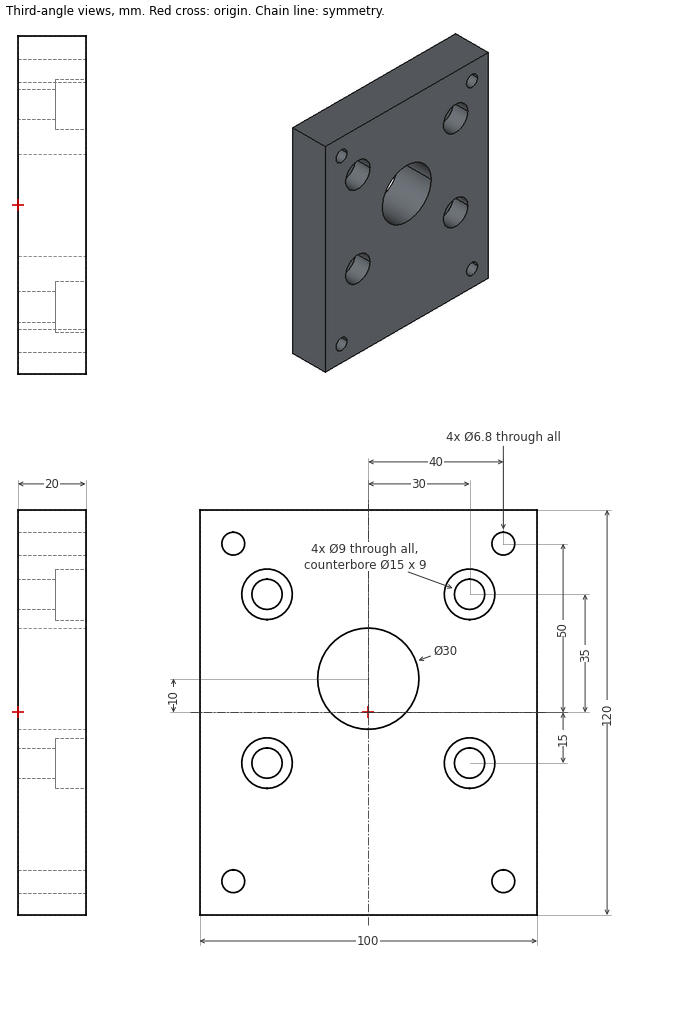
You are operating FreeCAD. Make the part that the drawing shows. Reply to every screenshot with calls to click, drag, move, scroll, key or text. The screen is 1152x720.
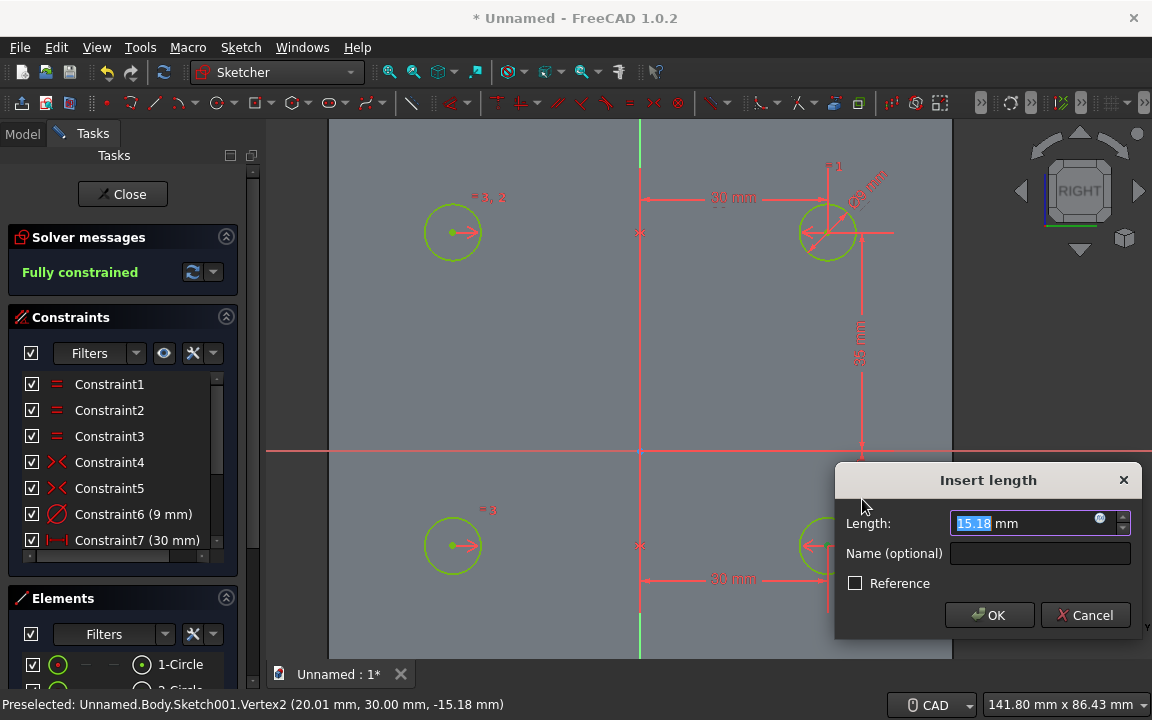
text(15)
key(Return)
key(Escape)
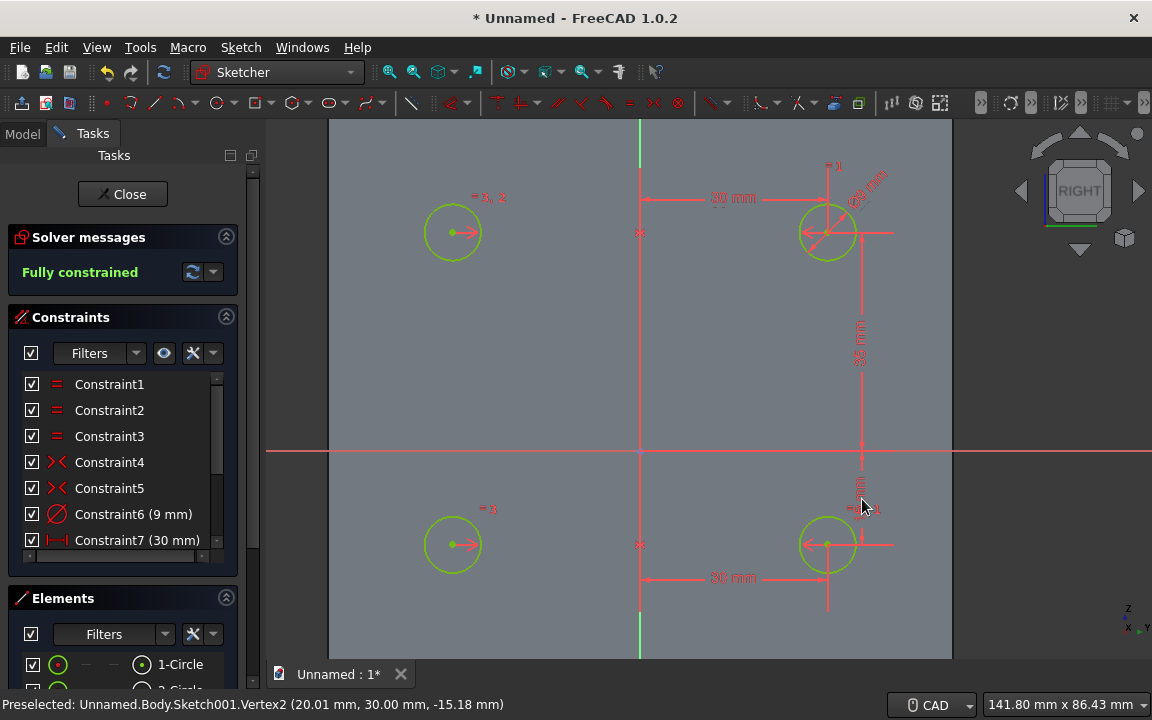
click(123, 194)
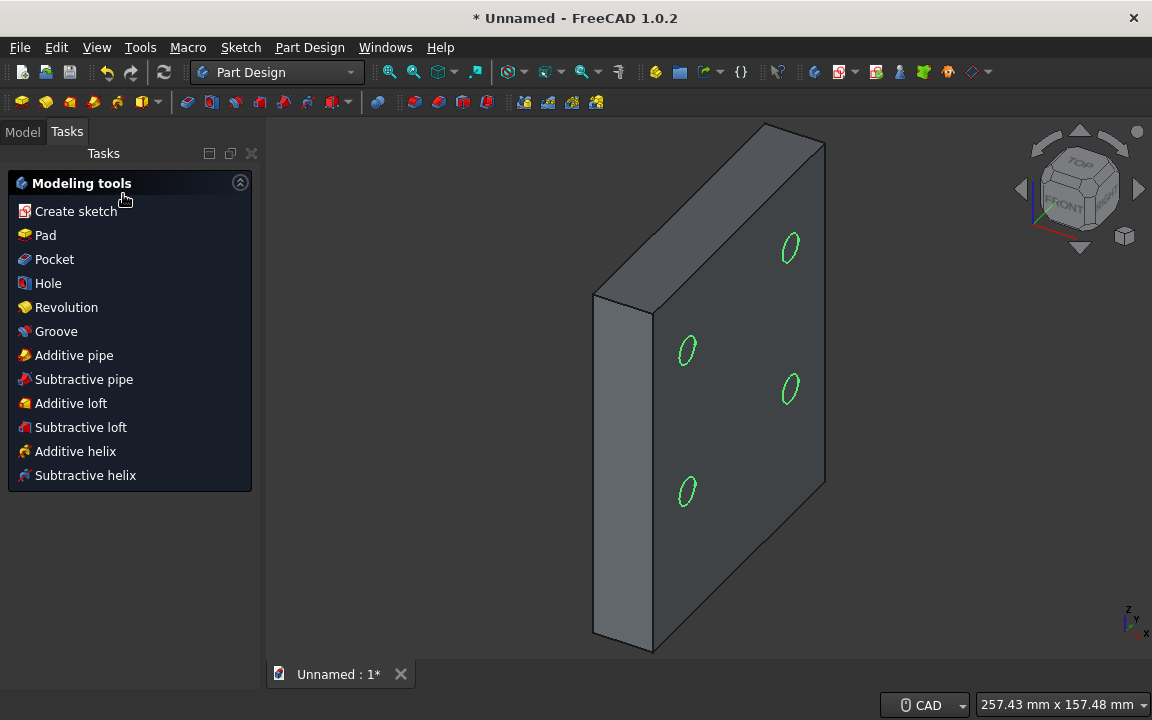
click(212, 102)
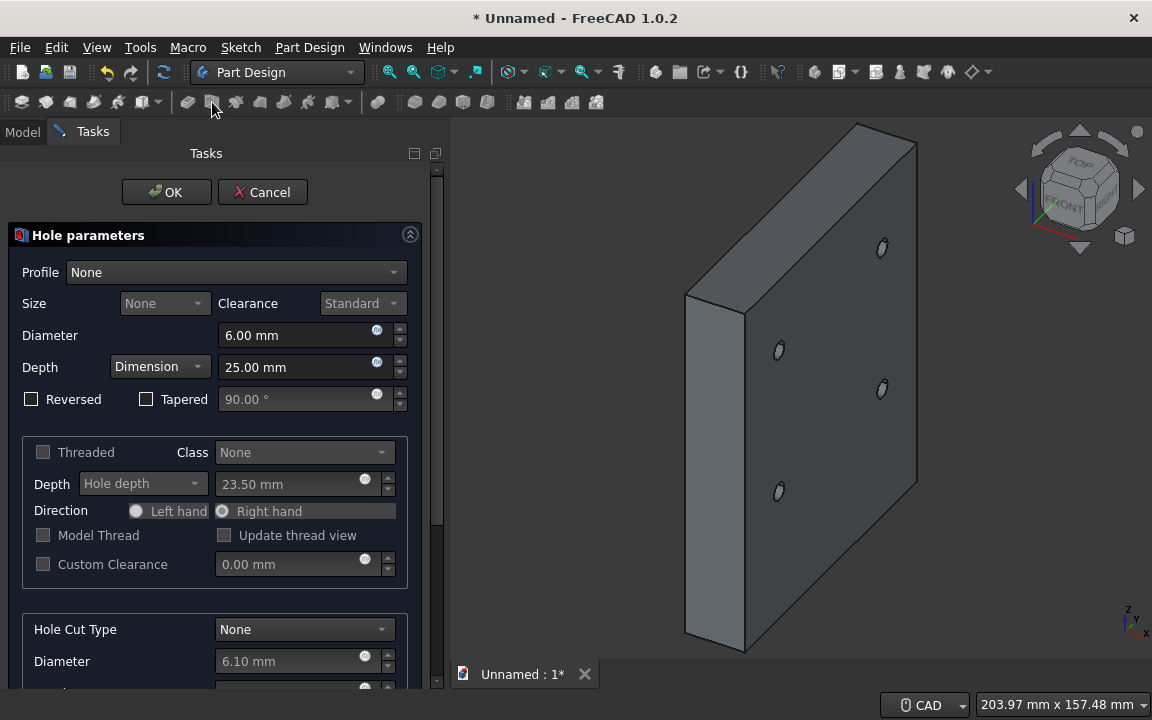
triple_click(305, 335)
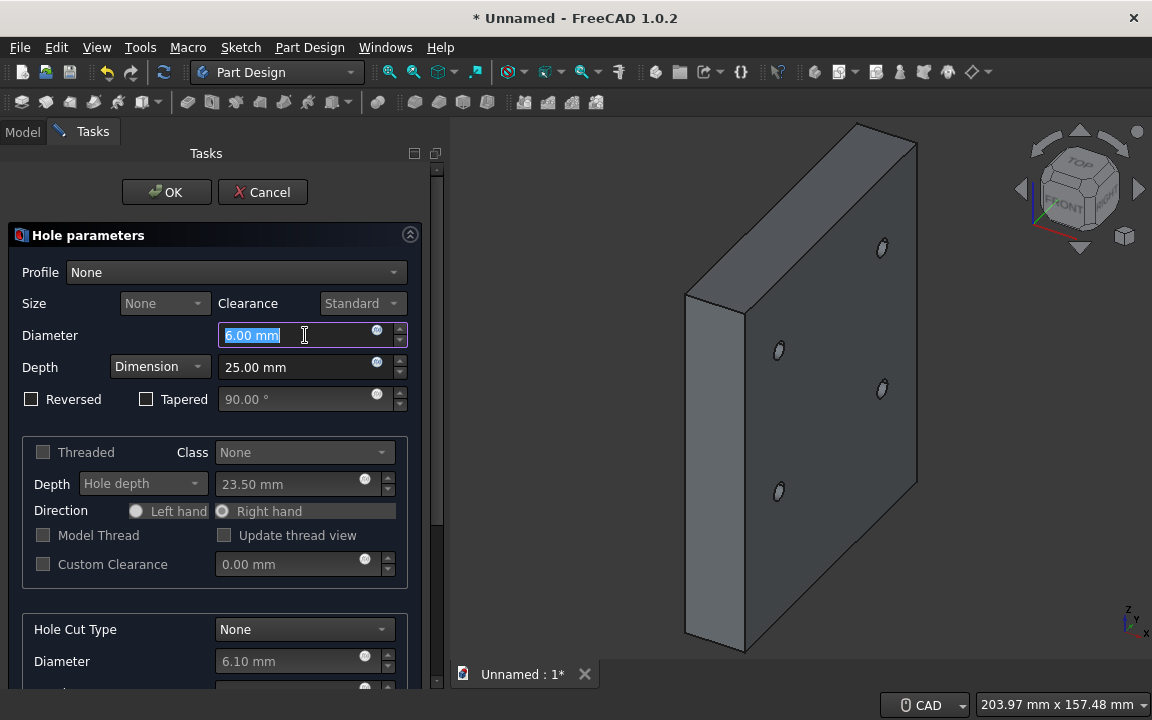
text(9)
key(Tab)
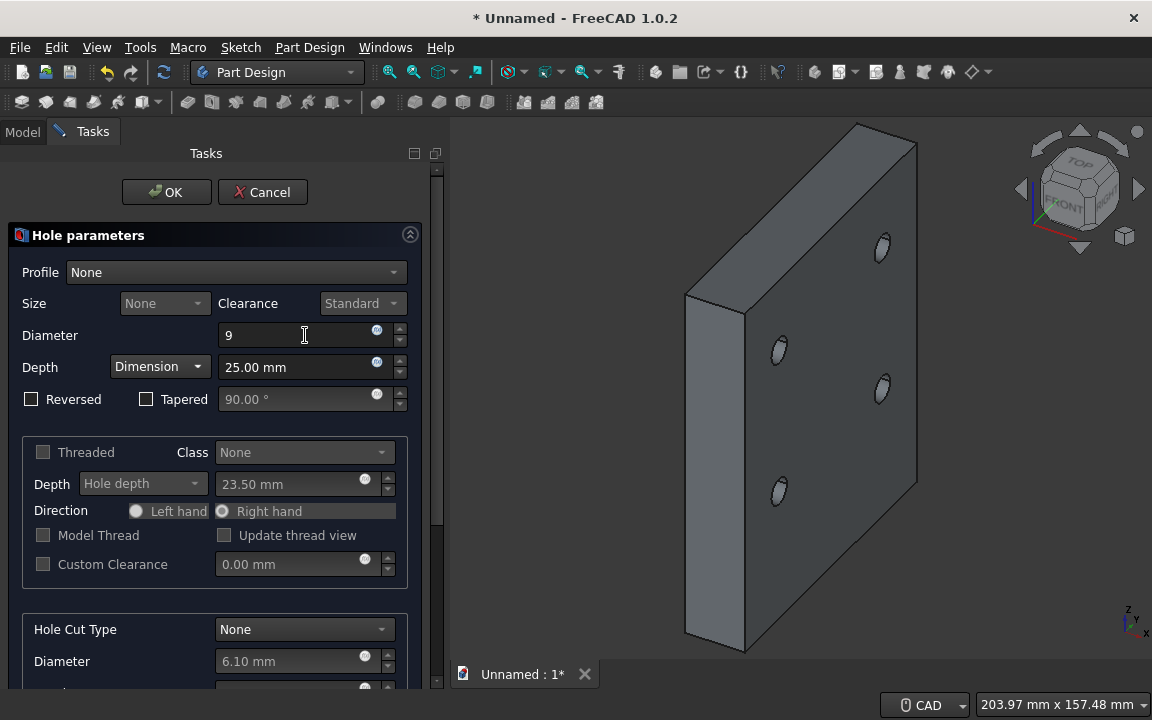
click(161, 366)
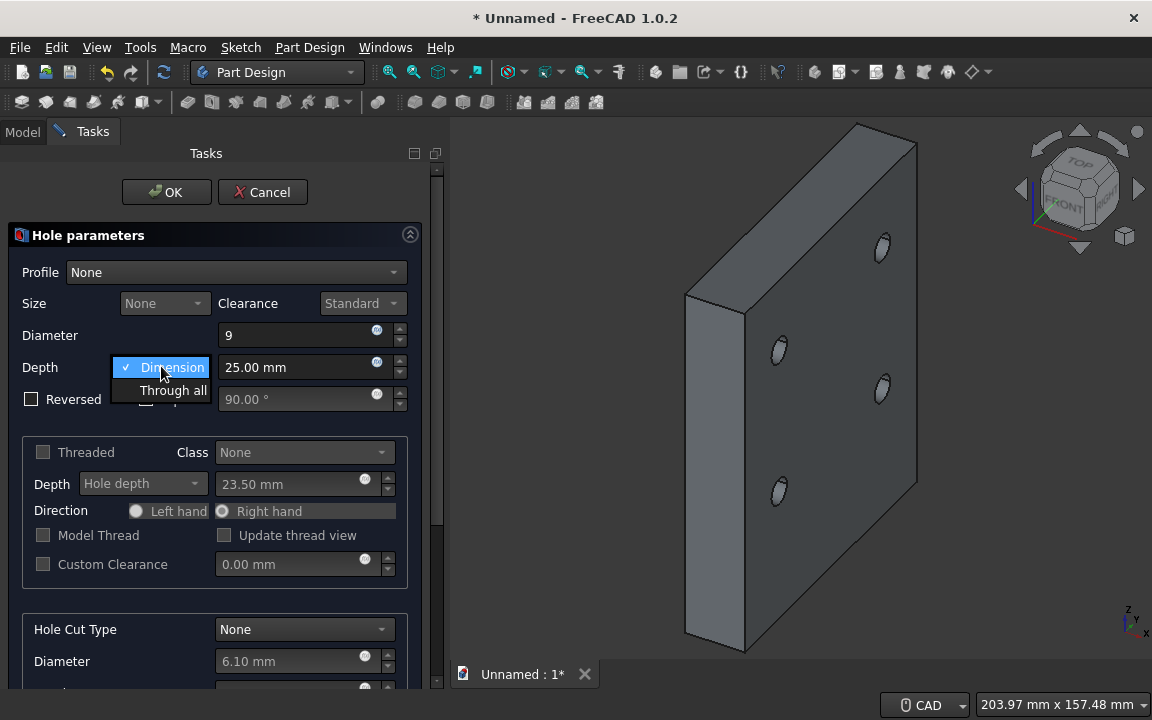
click(160, 390)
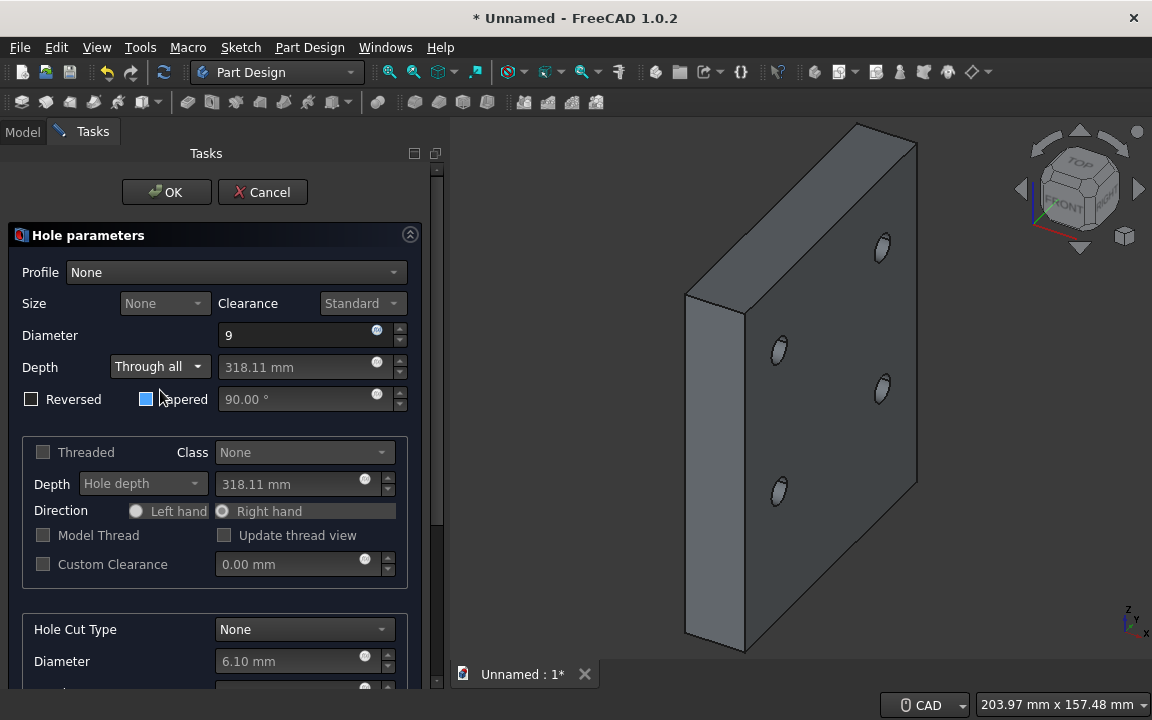
click(306, 630)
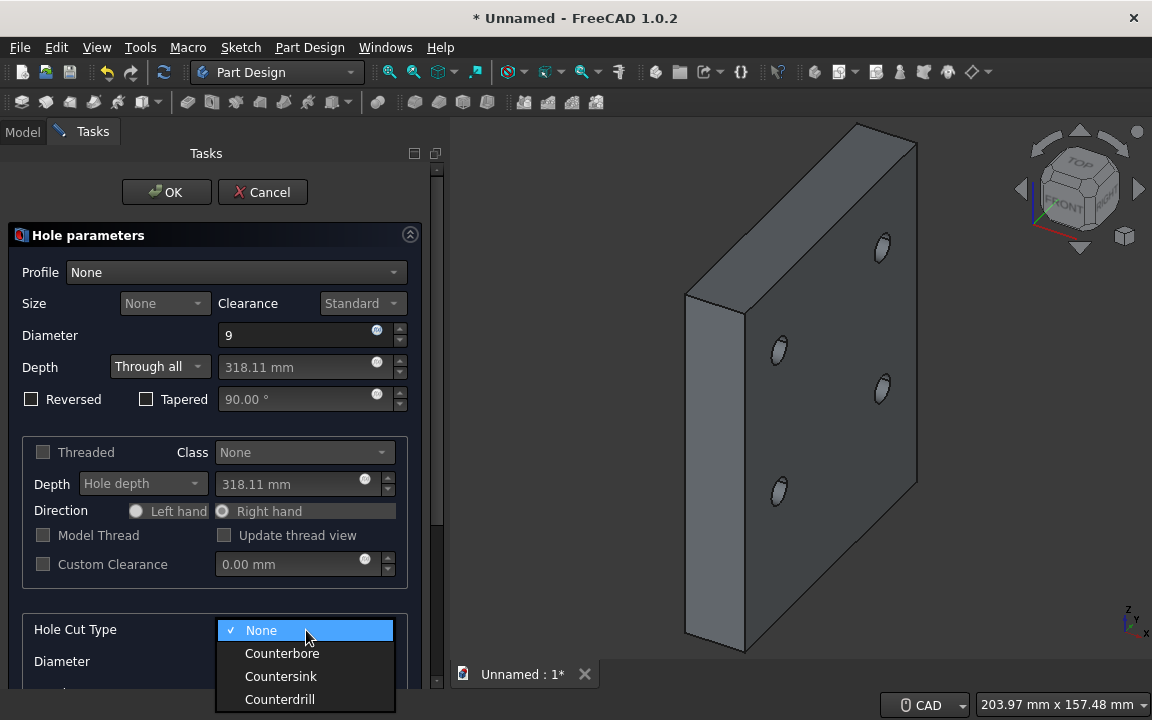
click(304, 654)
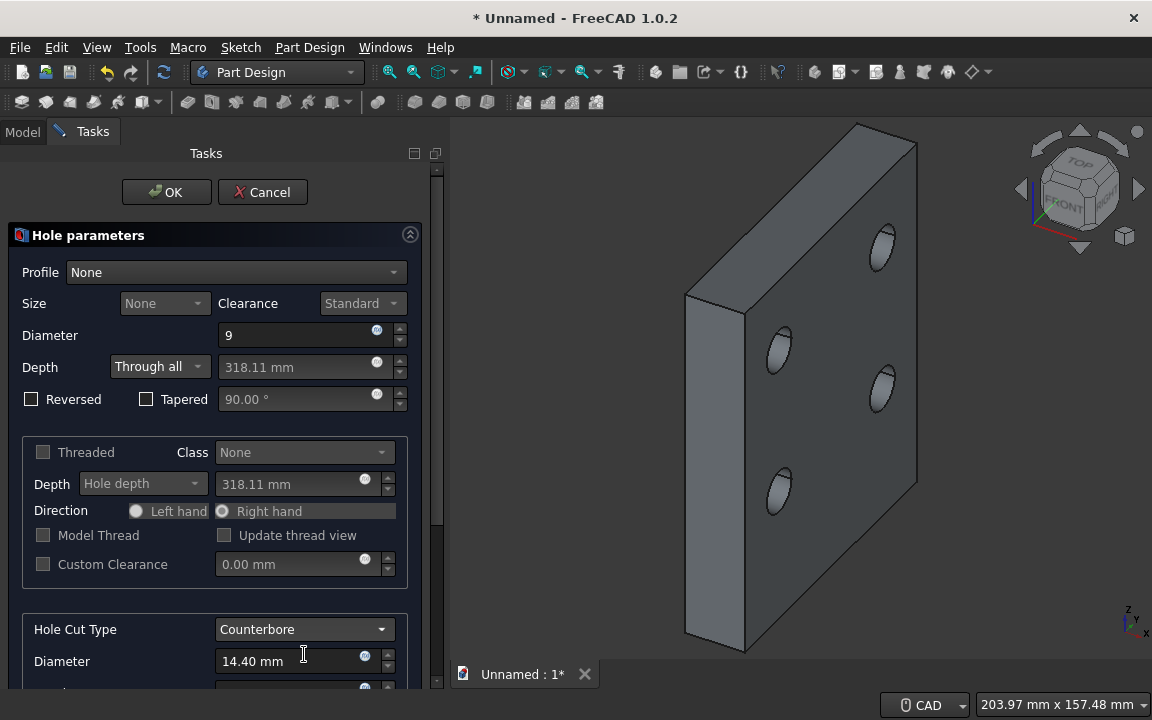
triple_click(298, 661)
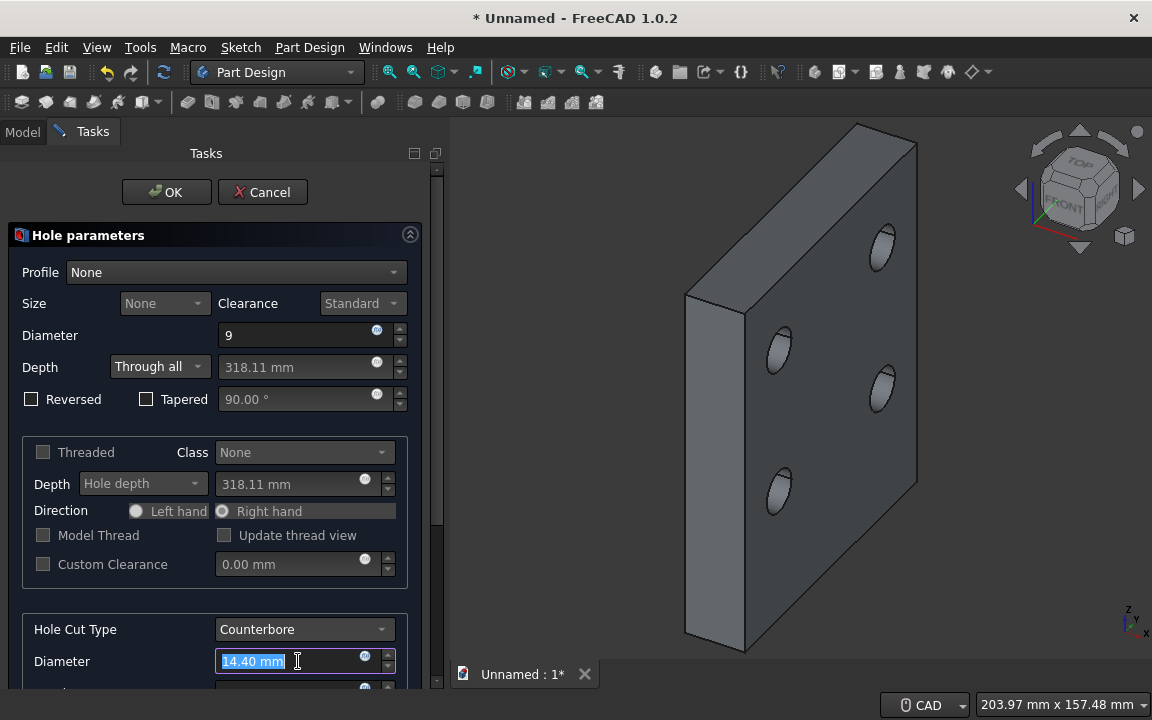
text(15)
key(Tab)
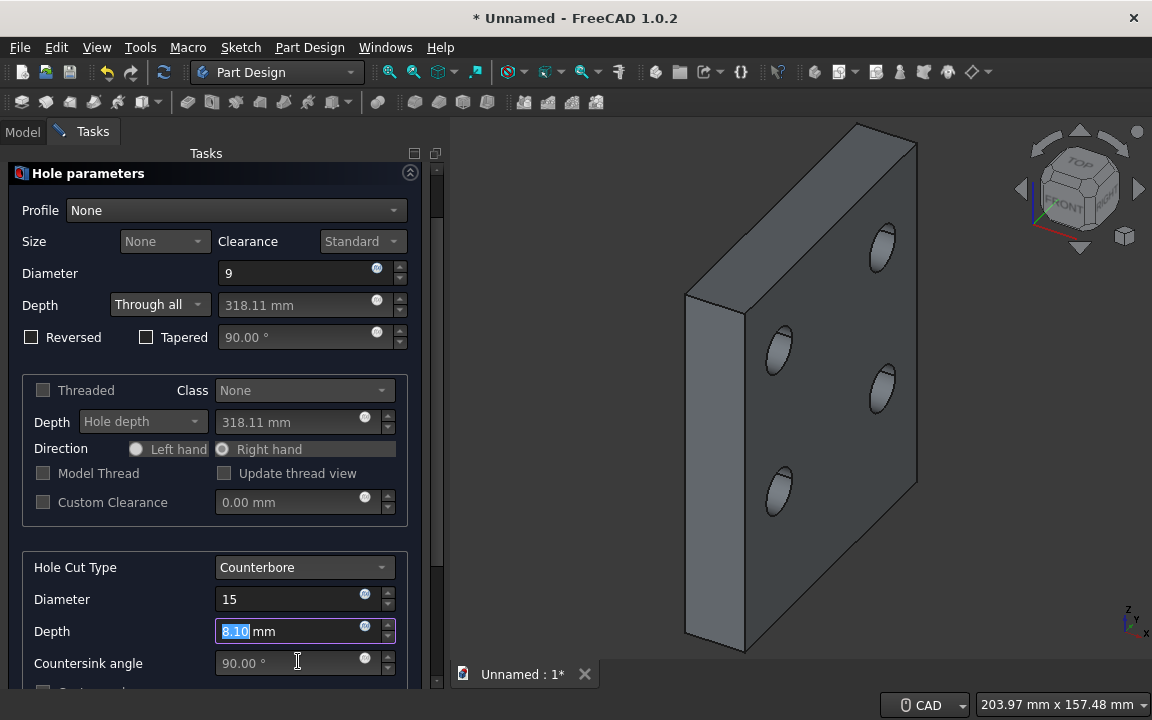
text(9)
key(Tab)